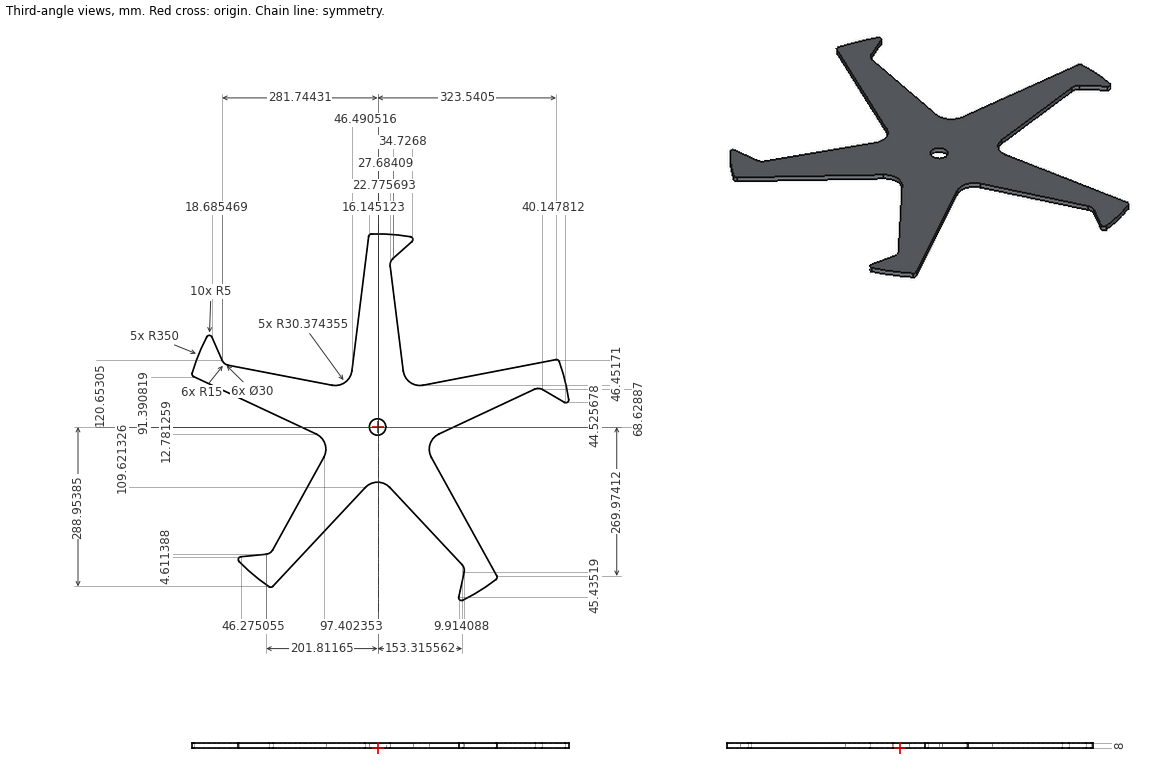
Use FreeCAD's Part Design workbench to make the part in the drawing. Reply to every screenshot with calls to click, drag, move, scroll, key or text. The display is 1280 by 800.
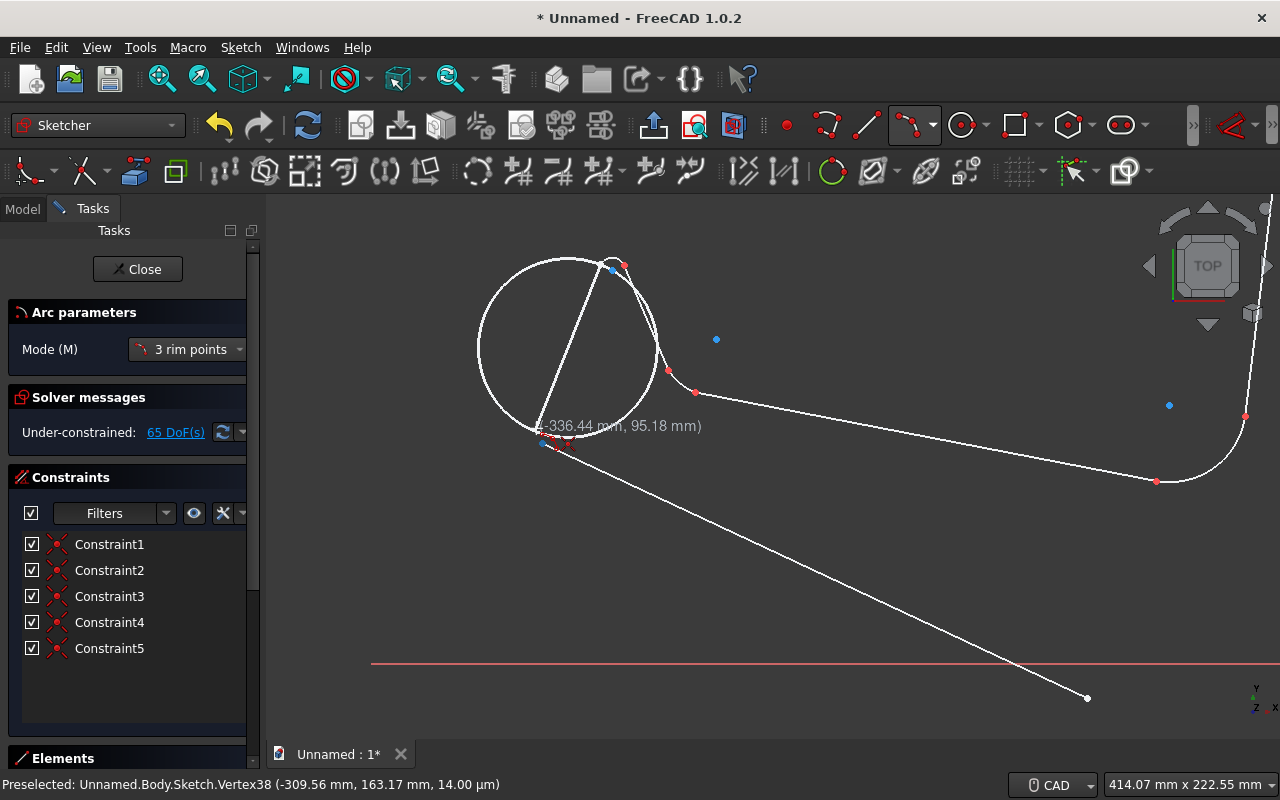
click(536, 426)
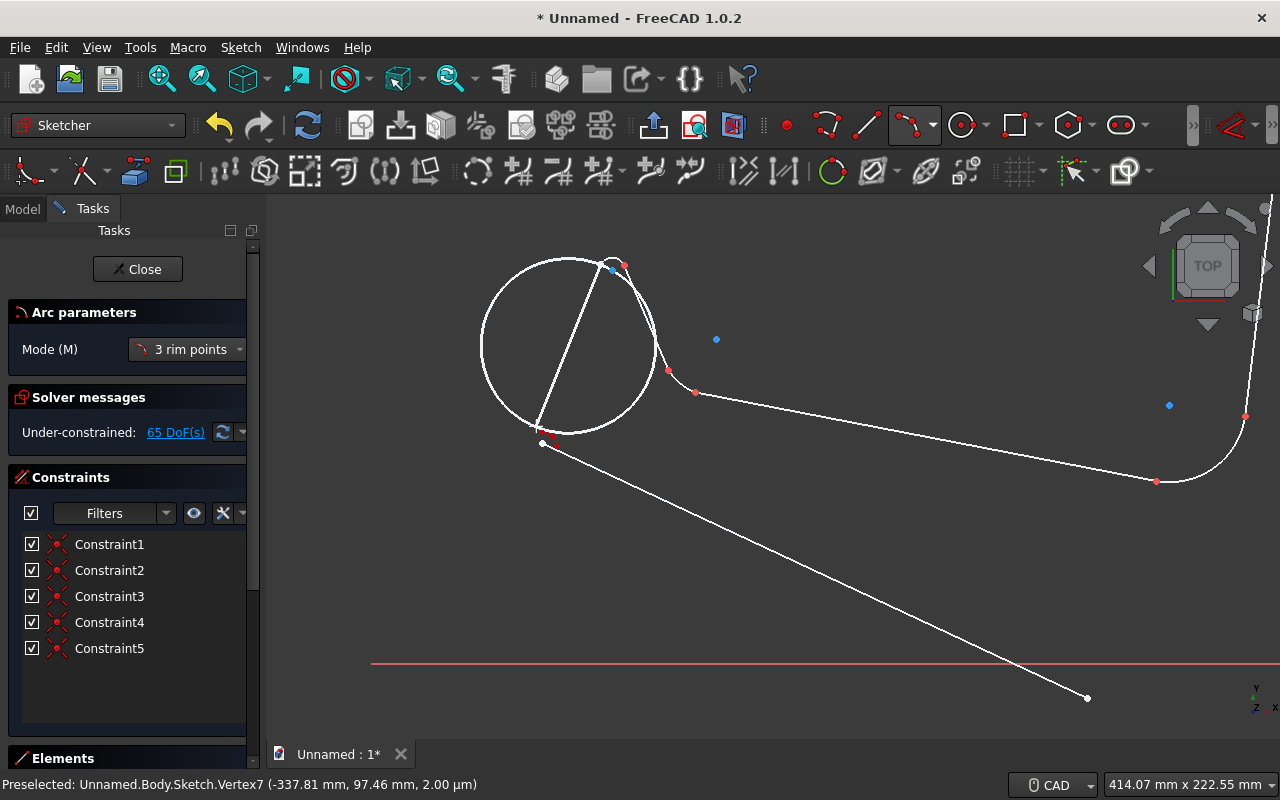
scroll(564, 343, up, 7)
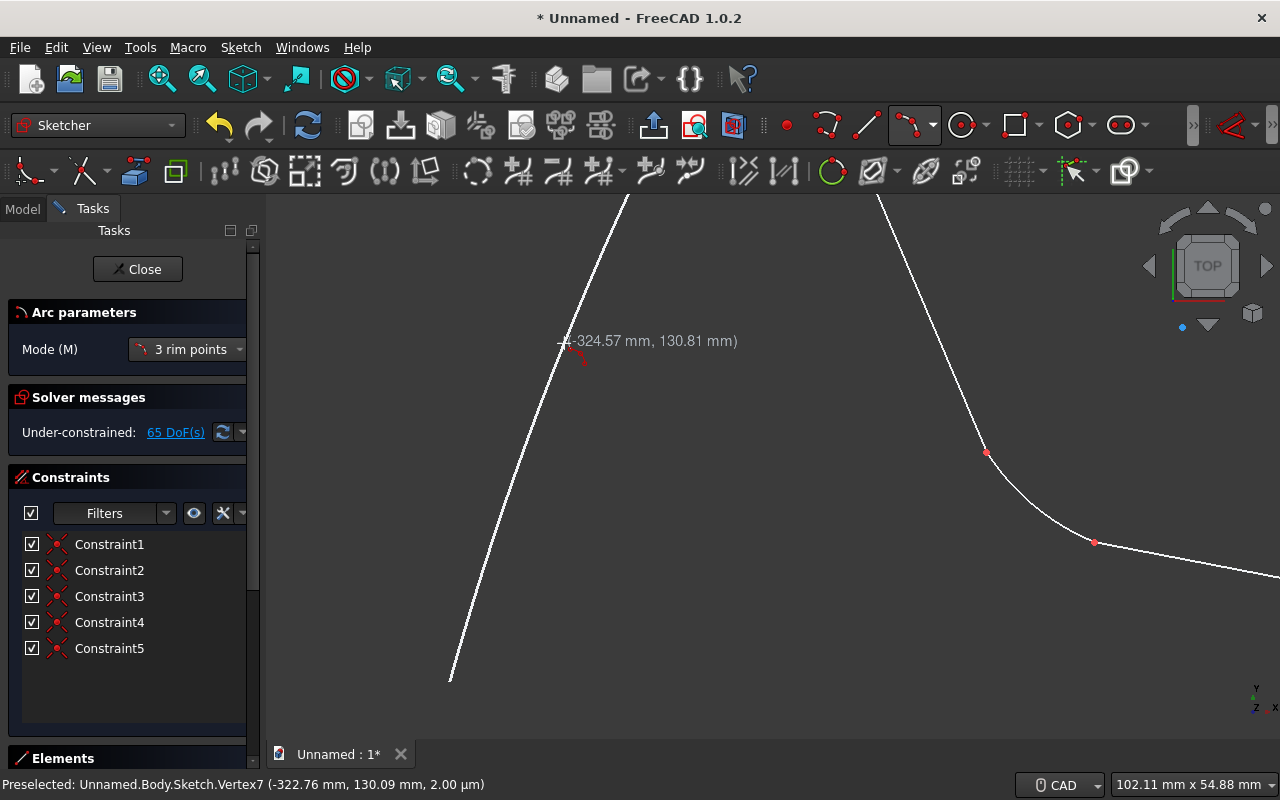
click(564, 343)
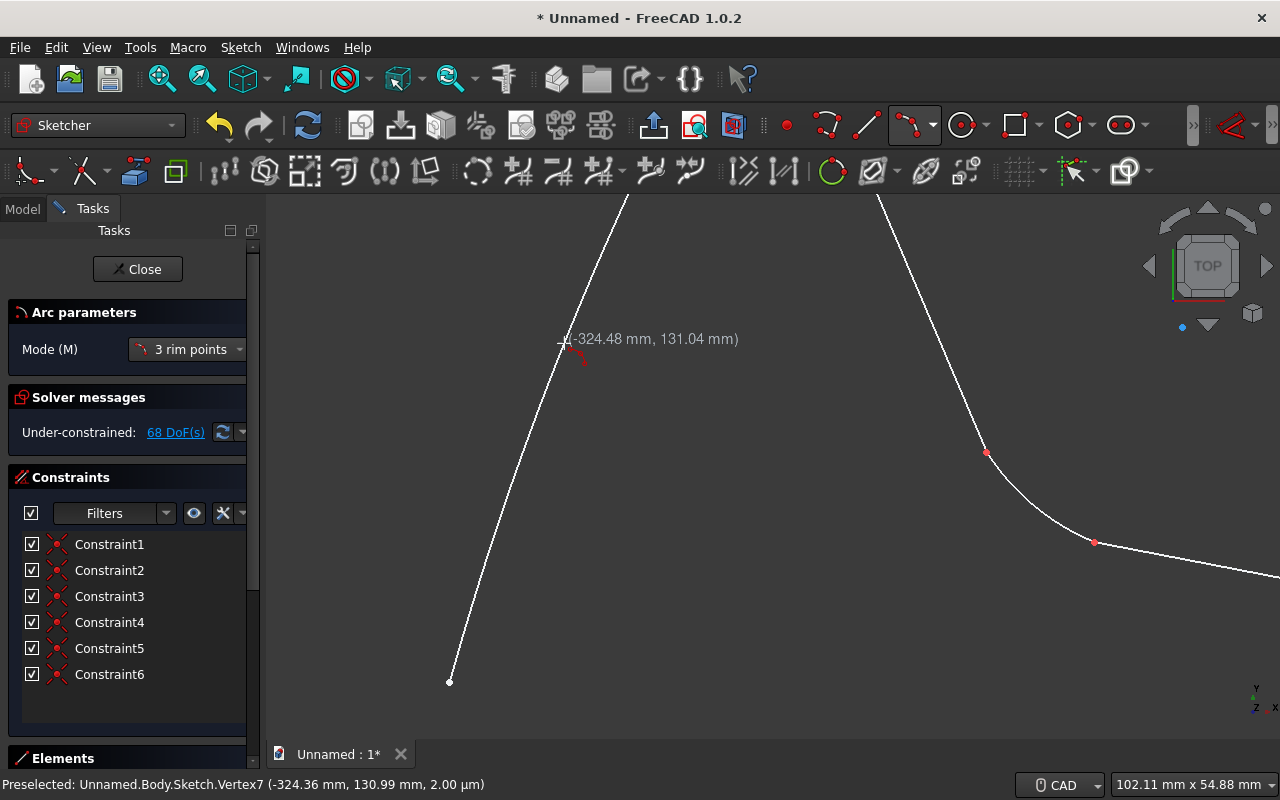
scroll(540, 414, down, 15)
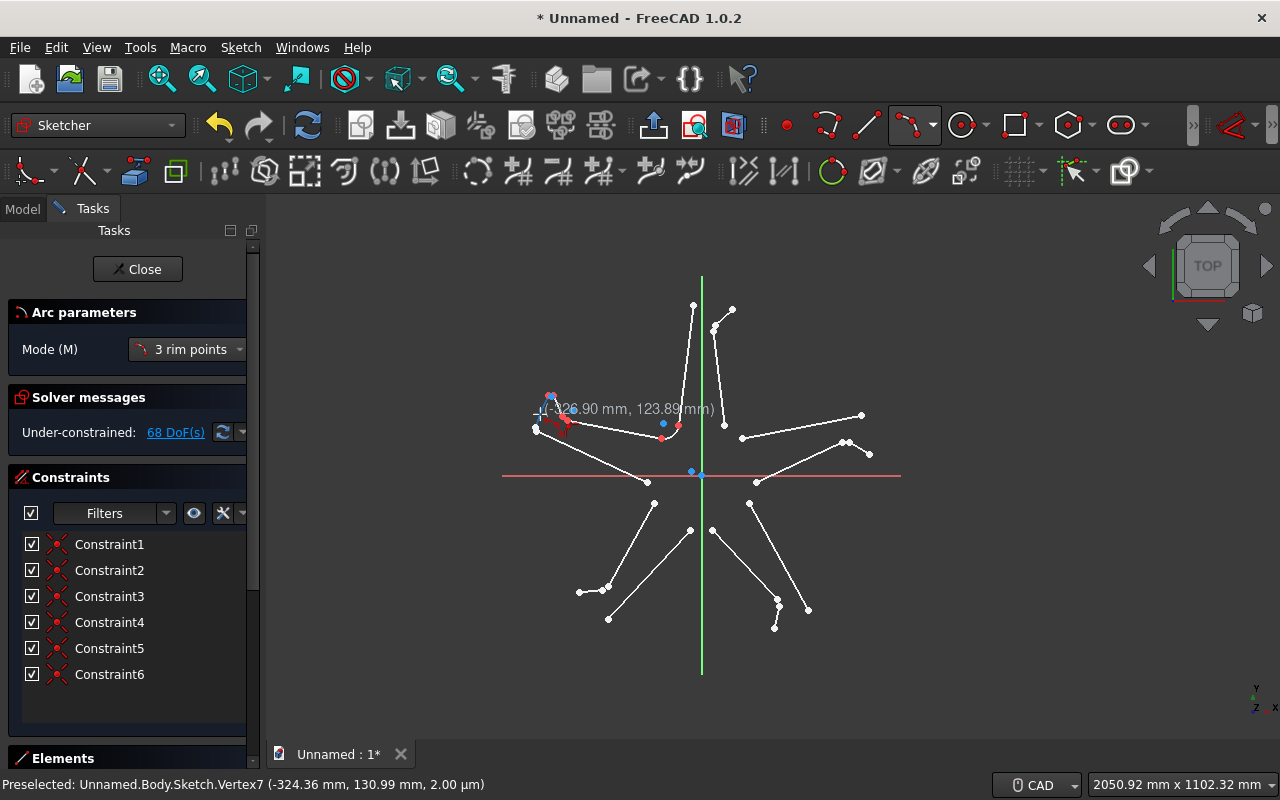
scroll(536, 428, up, 8)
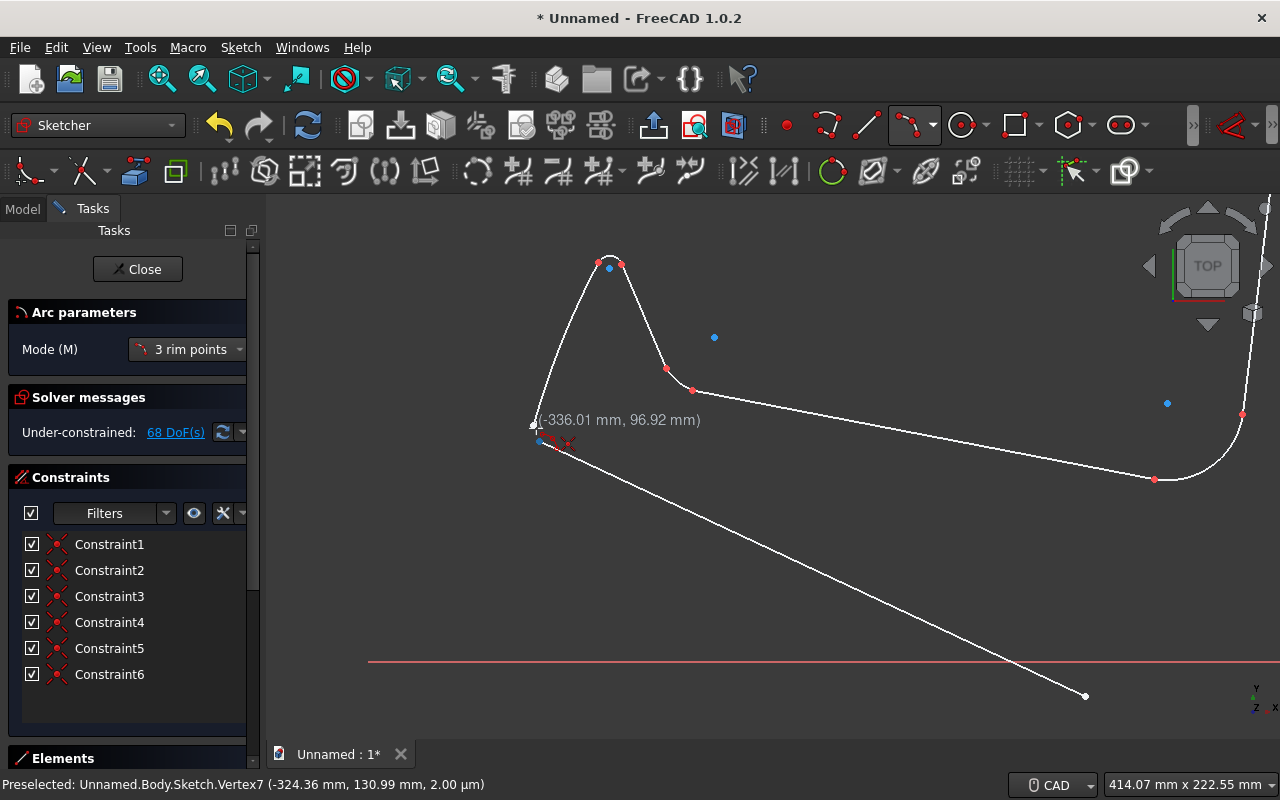
click(534, 425)
click(540, 441)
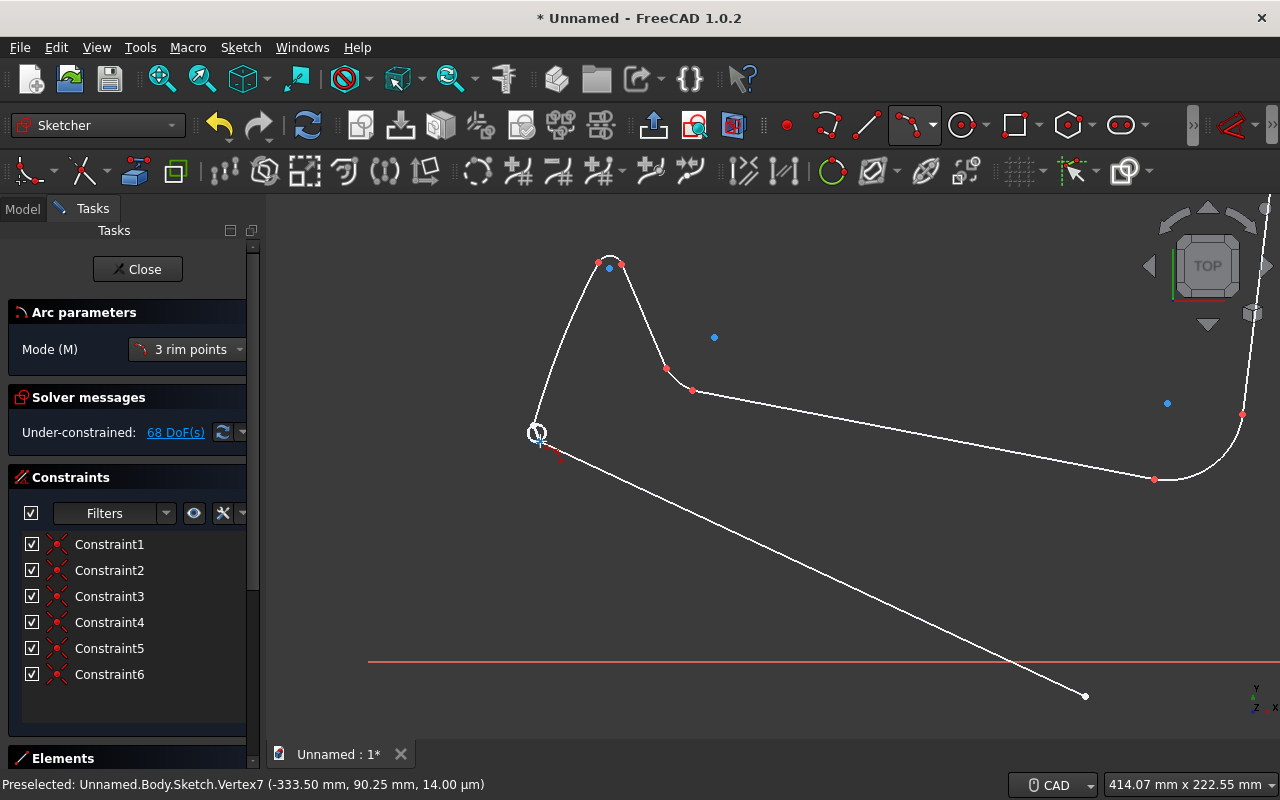
scroll(534, 433, up, 9)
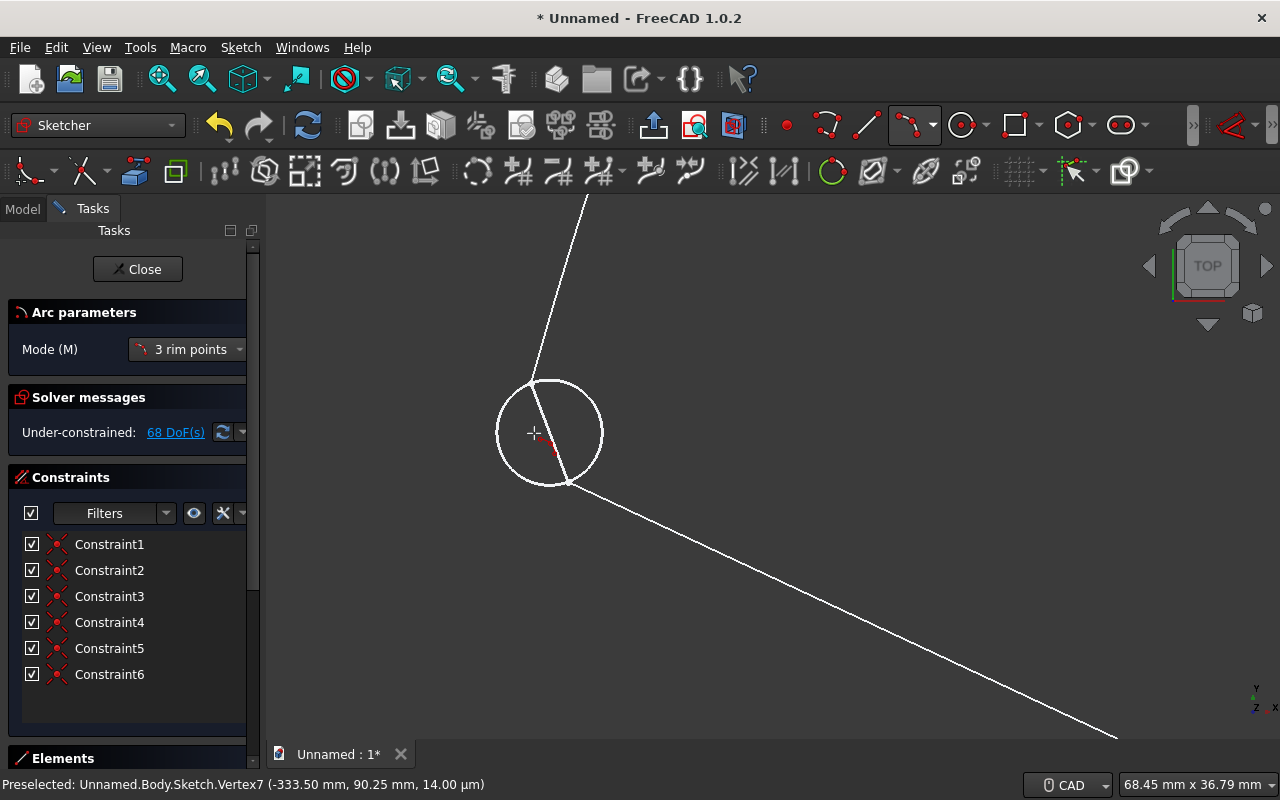
click(532, 429)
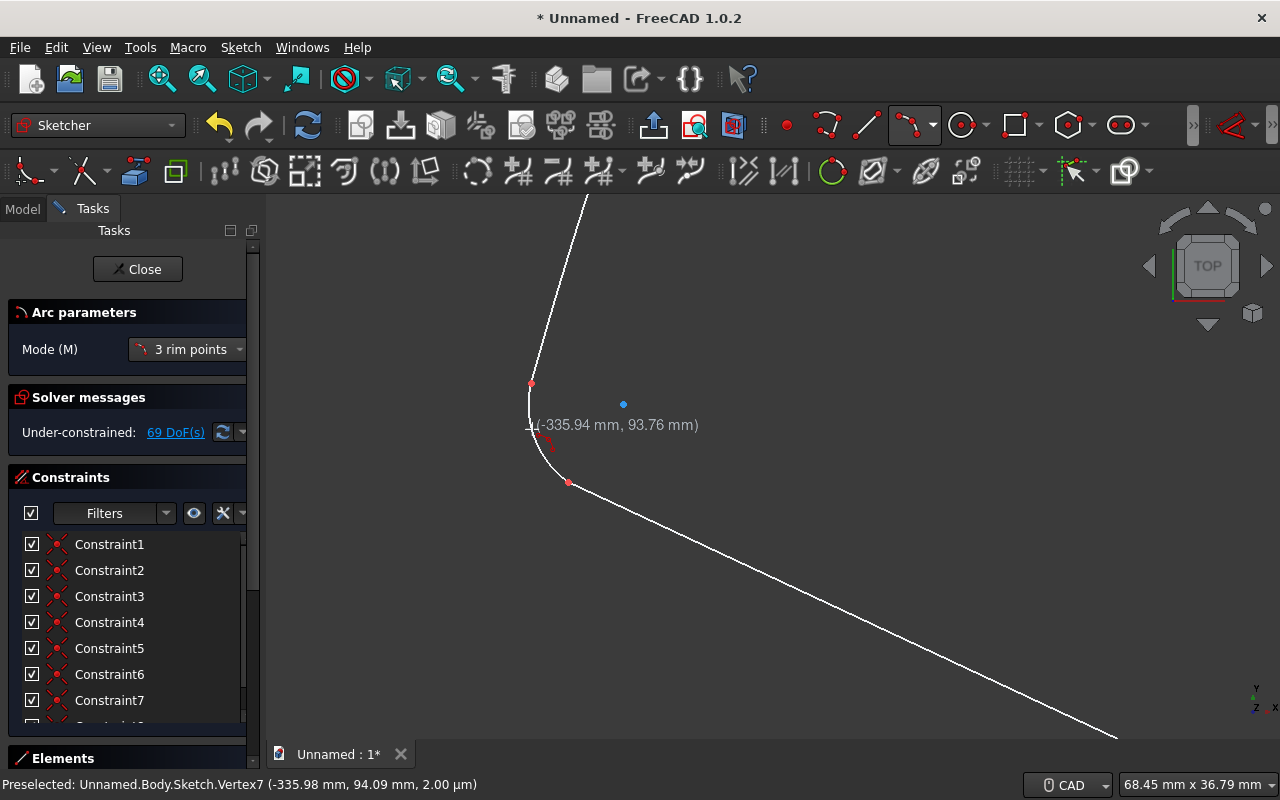
scroll(497, 420, down, 16)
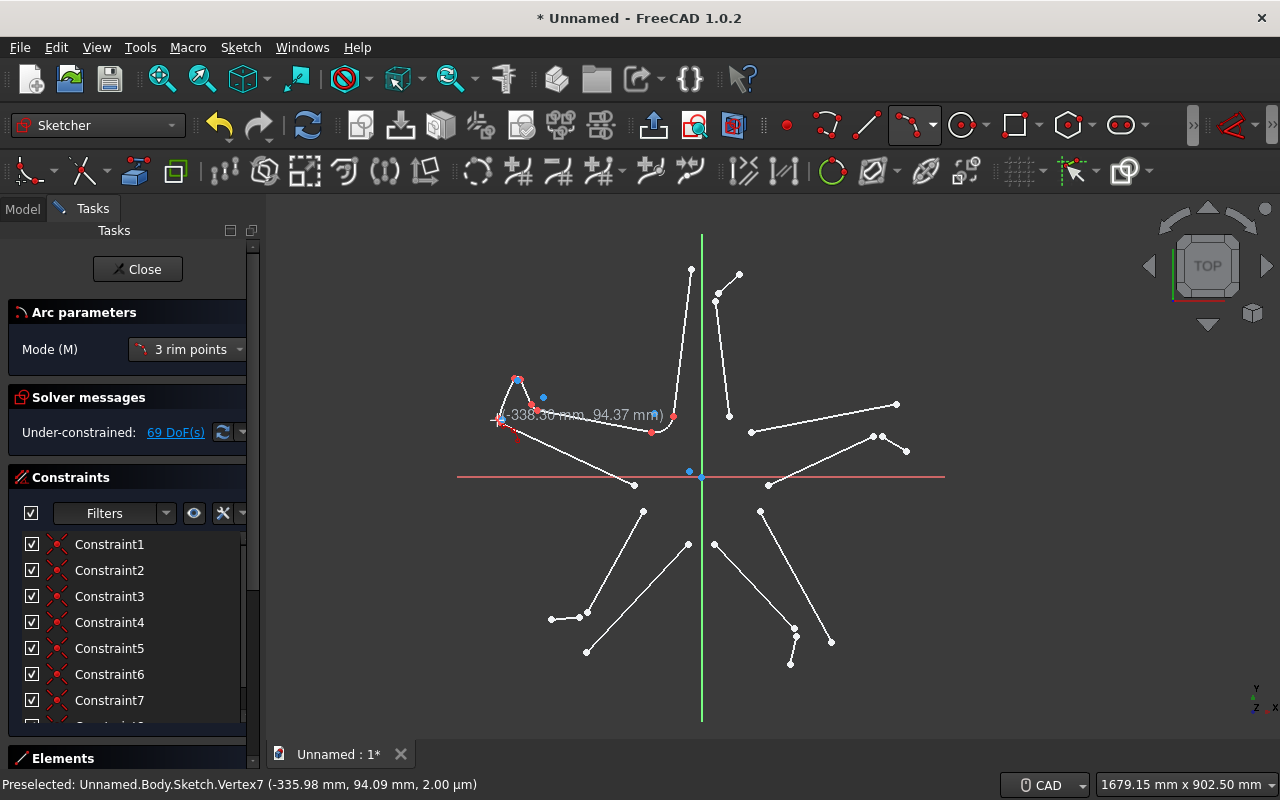
scroll(634, 485, up, 4)